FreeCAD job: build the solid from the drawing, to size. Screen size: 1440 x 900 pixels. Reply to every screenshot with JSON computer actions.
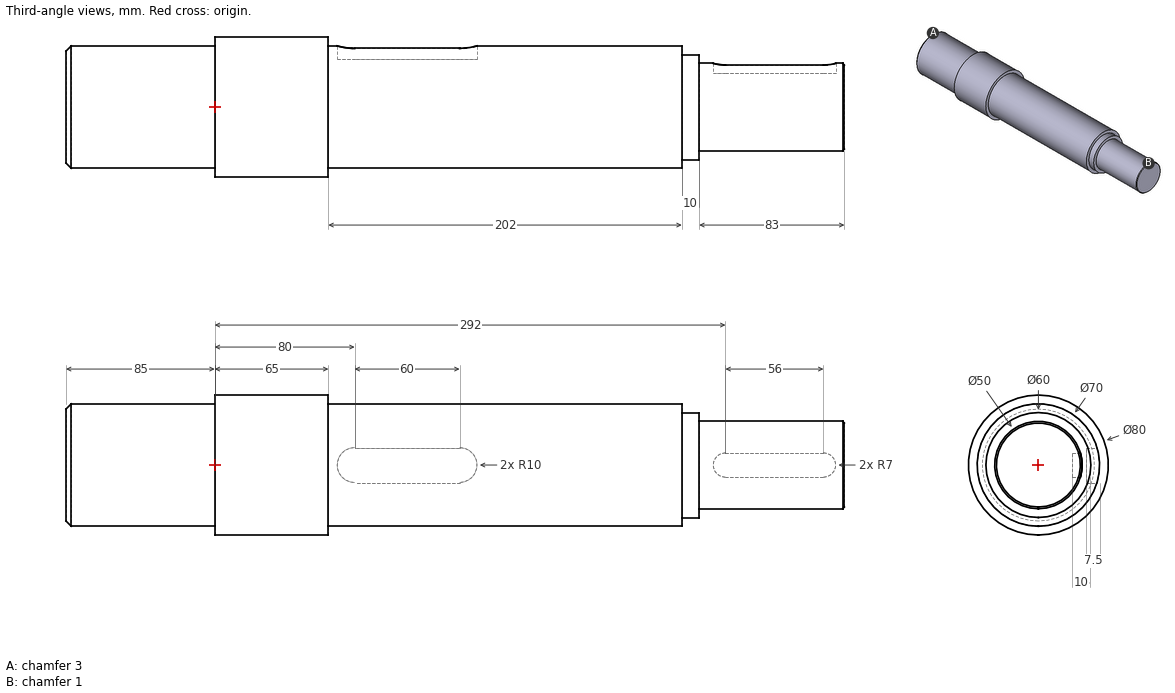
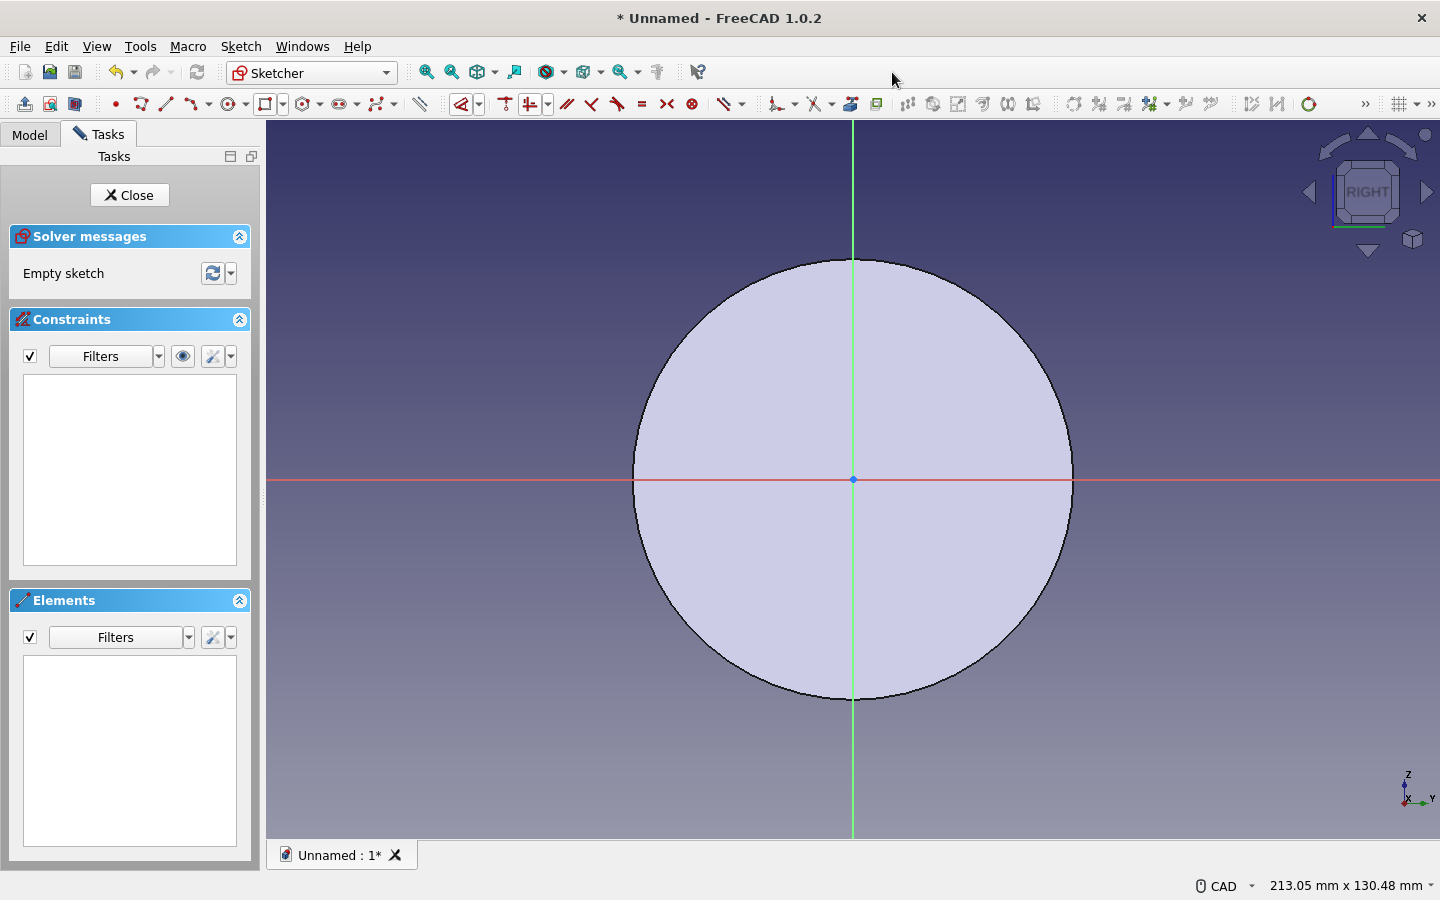
{"action": "key", "text": "g c"}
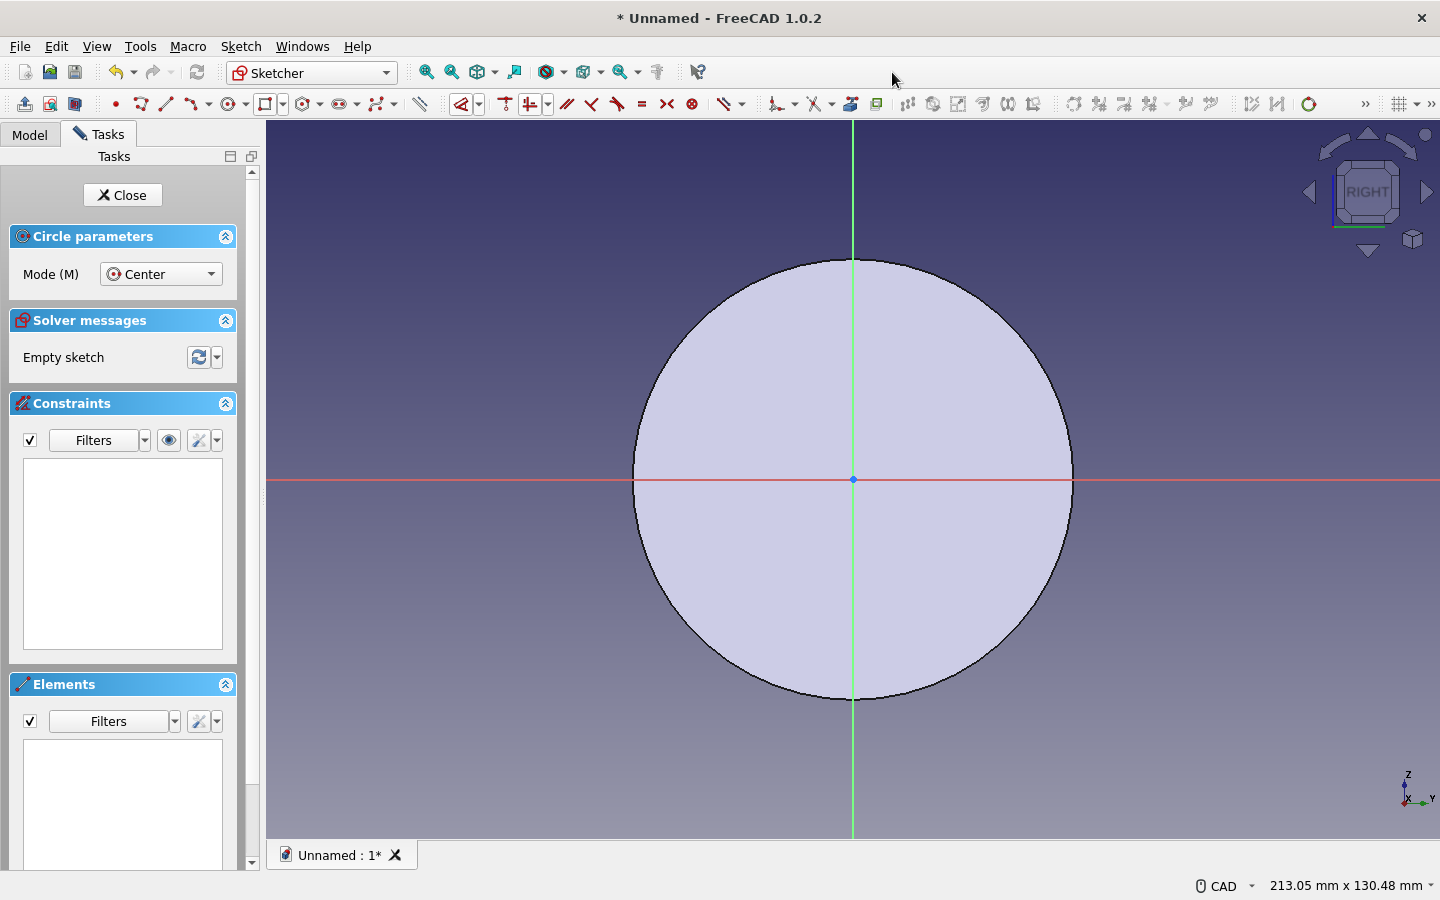
{"action": "left_click", "coordinate": [853, 479]}
{"action": "left_click", "coordinate": [989, 343]}
{"action": "key", "text": "Escape"}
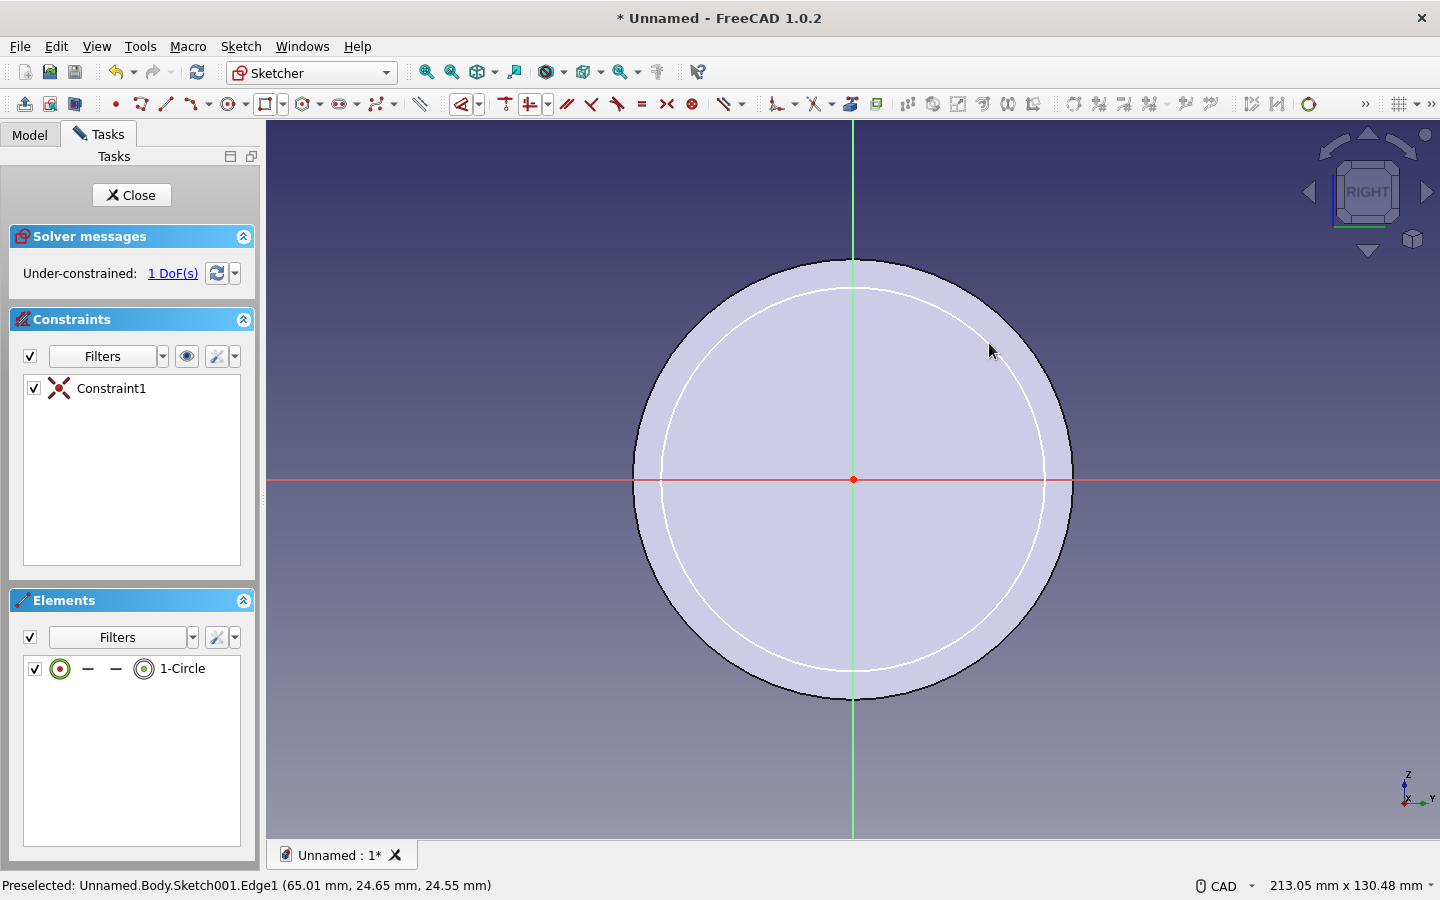
{"action": "key", "text": "d"}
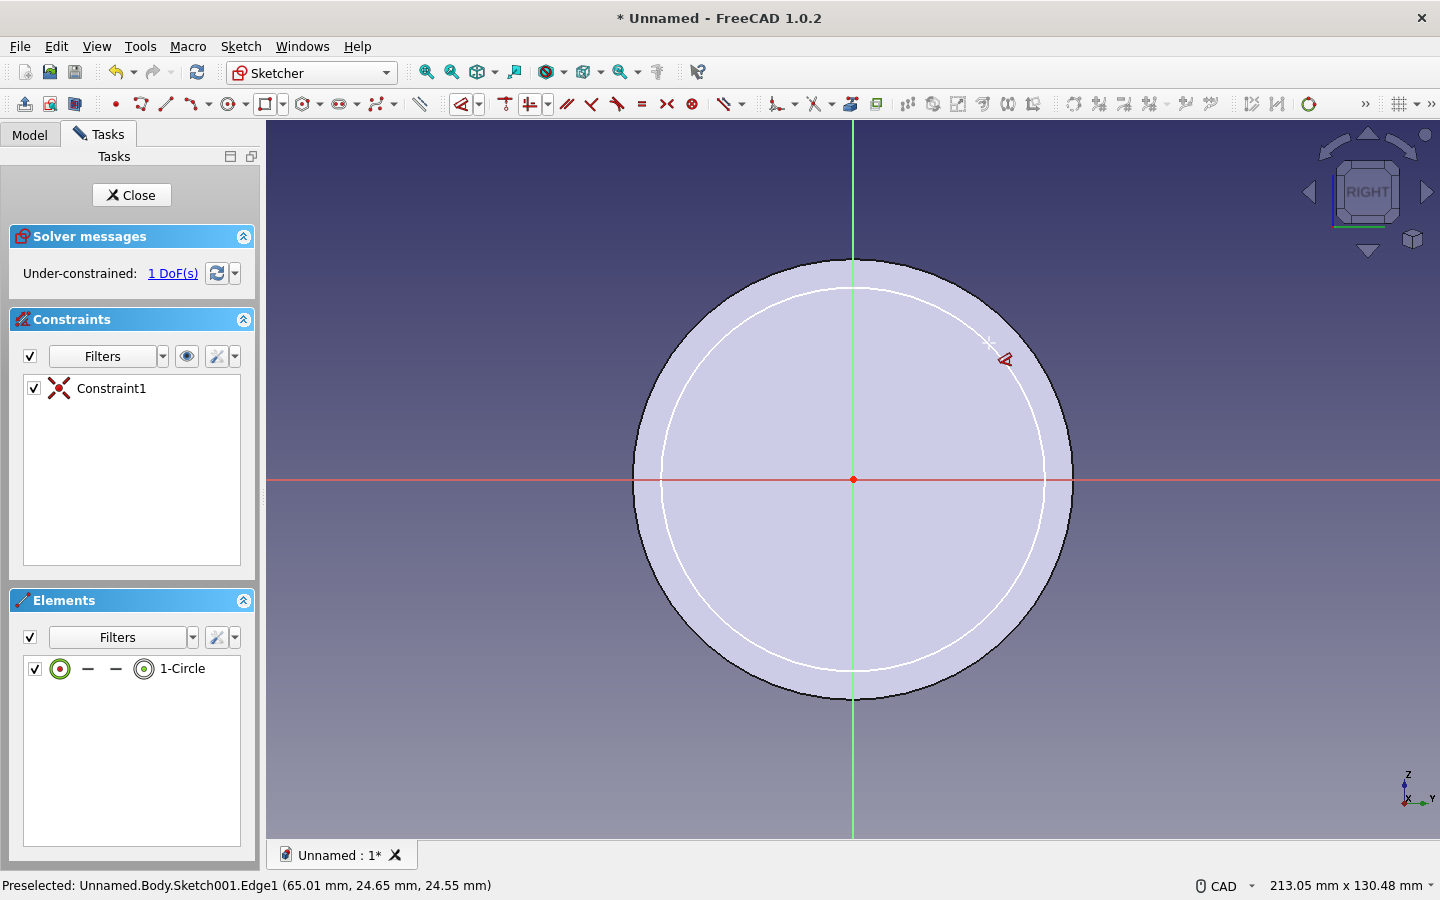
{"action": "left_click", "coordinate": [988, 343]}
{"action": "left_click", "coordinate": [1011, 320]}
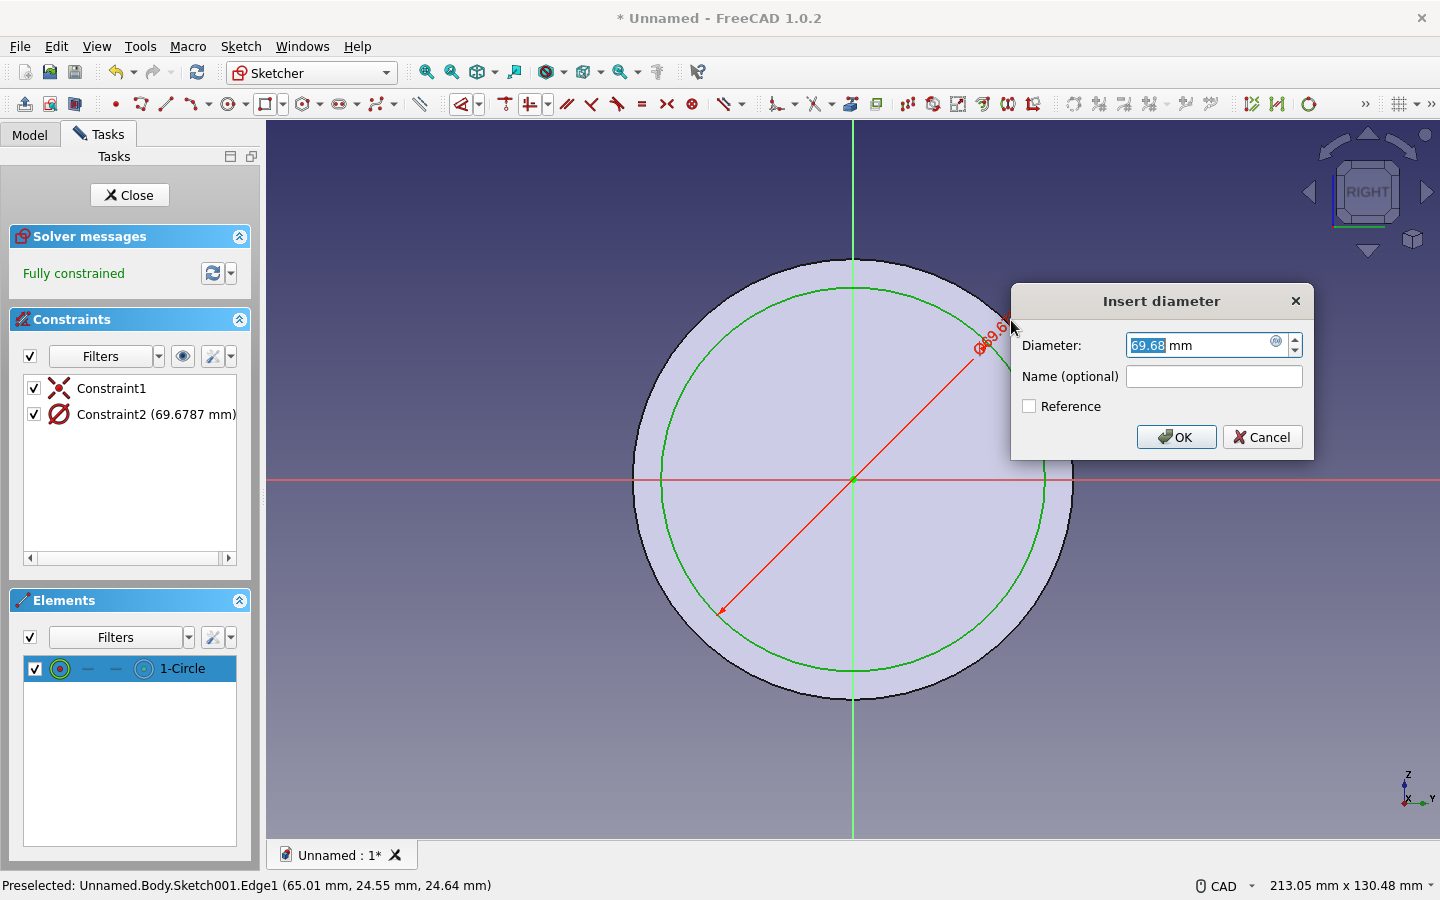
{"action": "type", "text": "70"}
{"action": "key", "text": "Return"}
{"action": "key", "text": "Escape"}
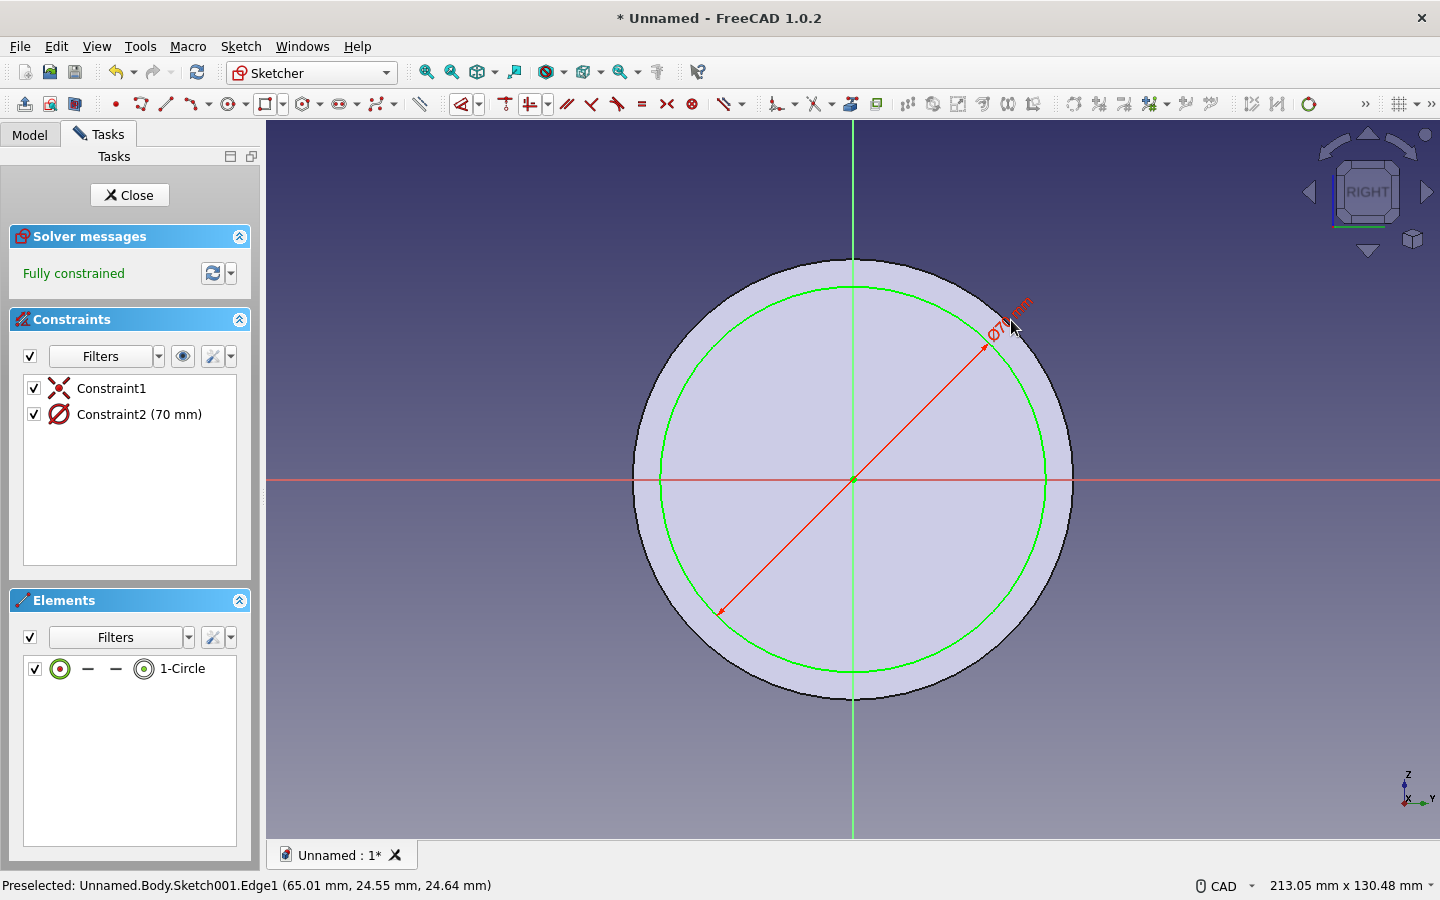
{"action": "left_click", "coordinate": [130, 195]}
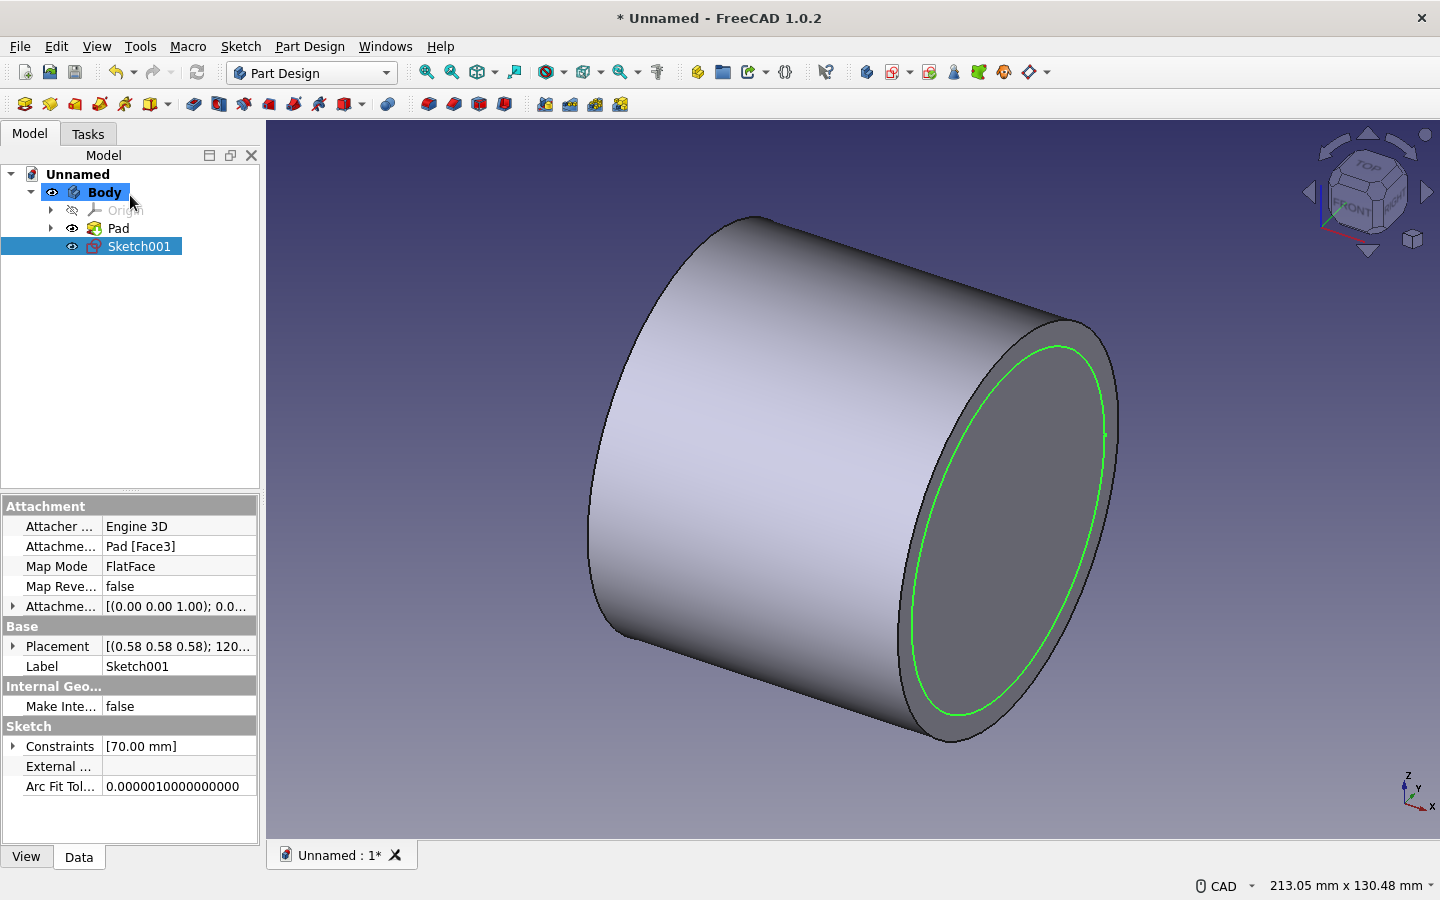
{"action": "left_click", "coordinate": [25, 104]}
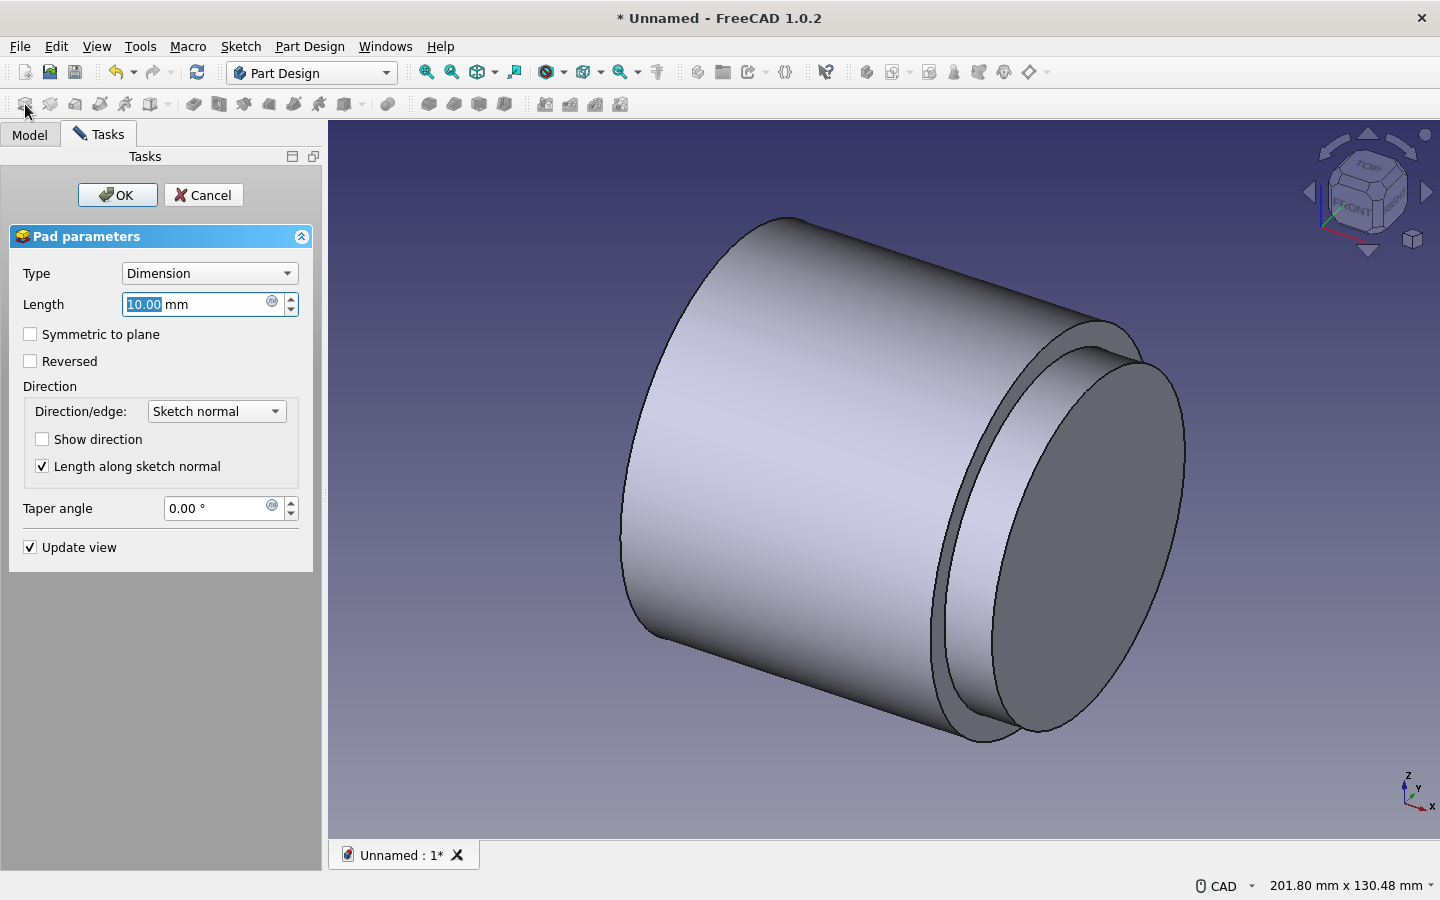
{"action": "type", "text": "202"}
{"action": "key", "text": "Tab"}